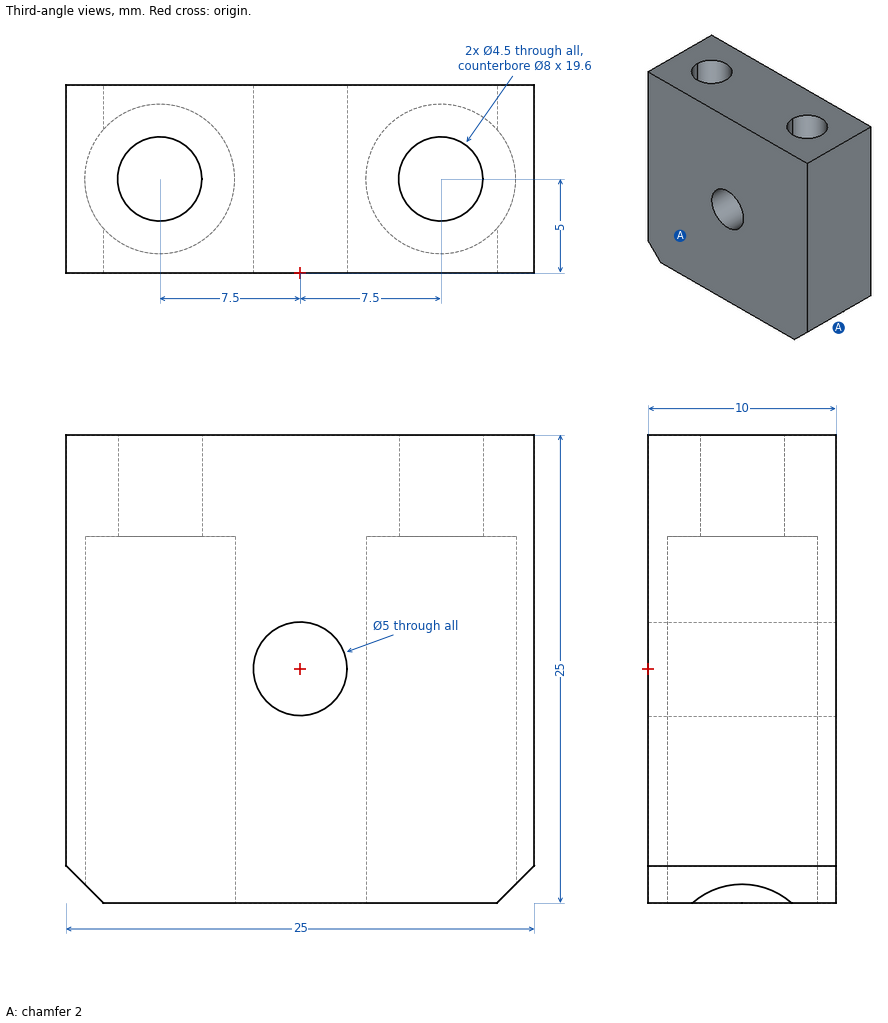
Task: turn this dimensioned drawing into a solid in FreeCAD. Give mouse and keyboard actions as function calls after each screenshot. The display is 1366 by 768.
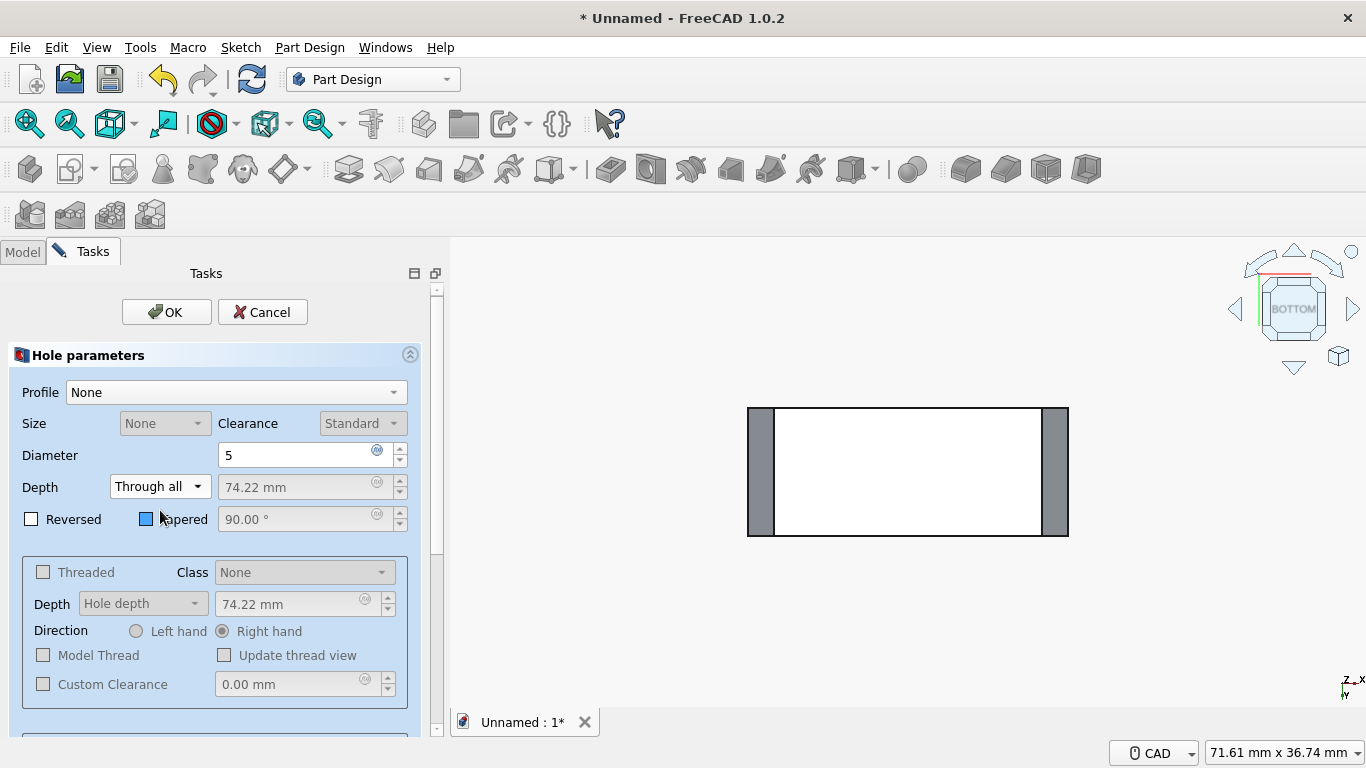
click(167, 312)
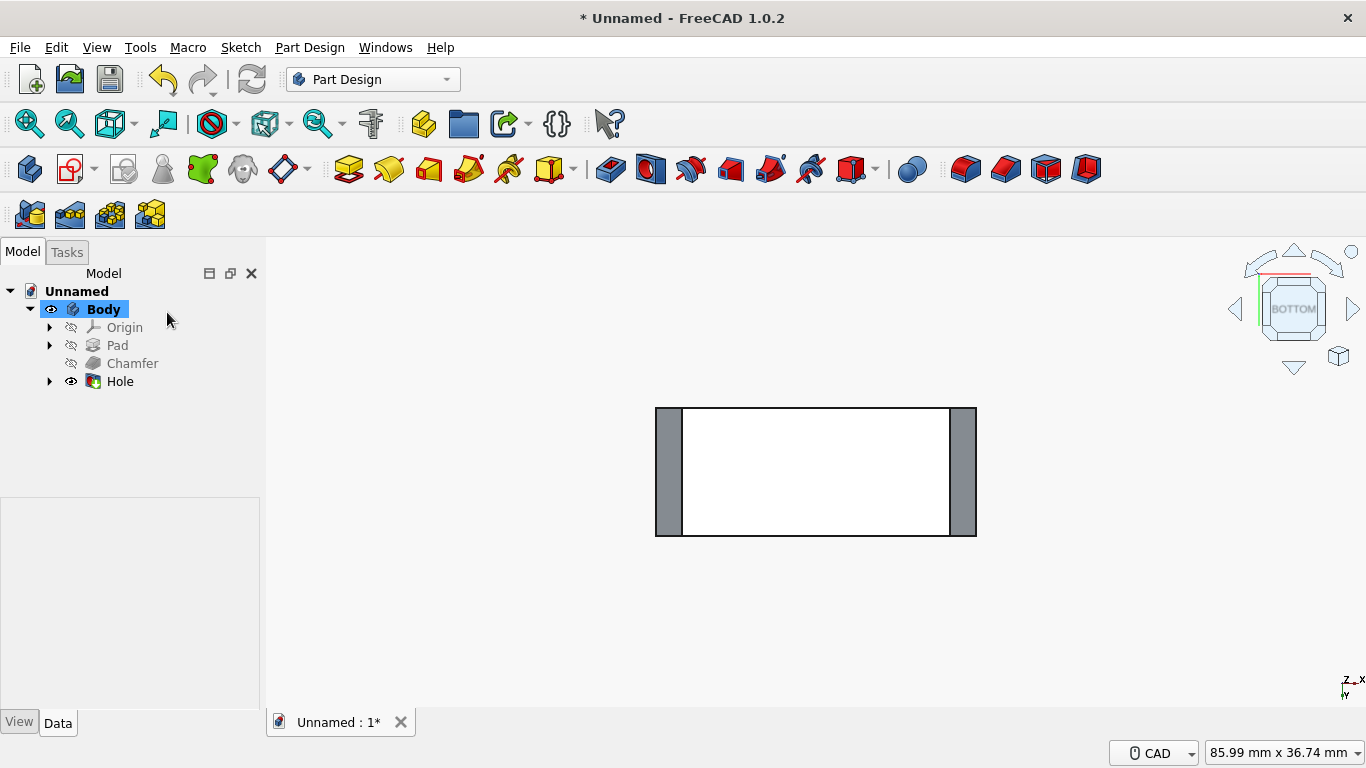
click(30, 124)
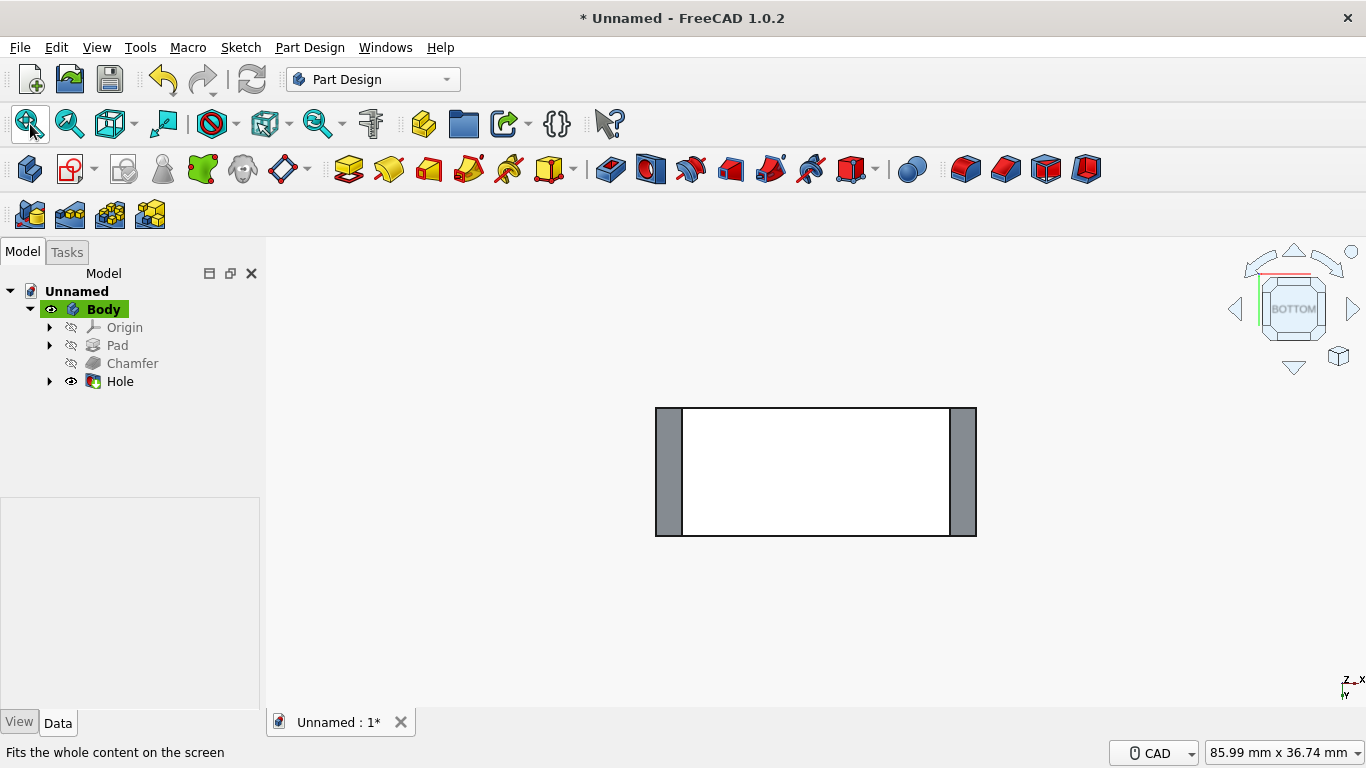
click(854, 471)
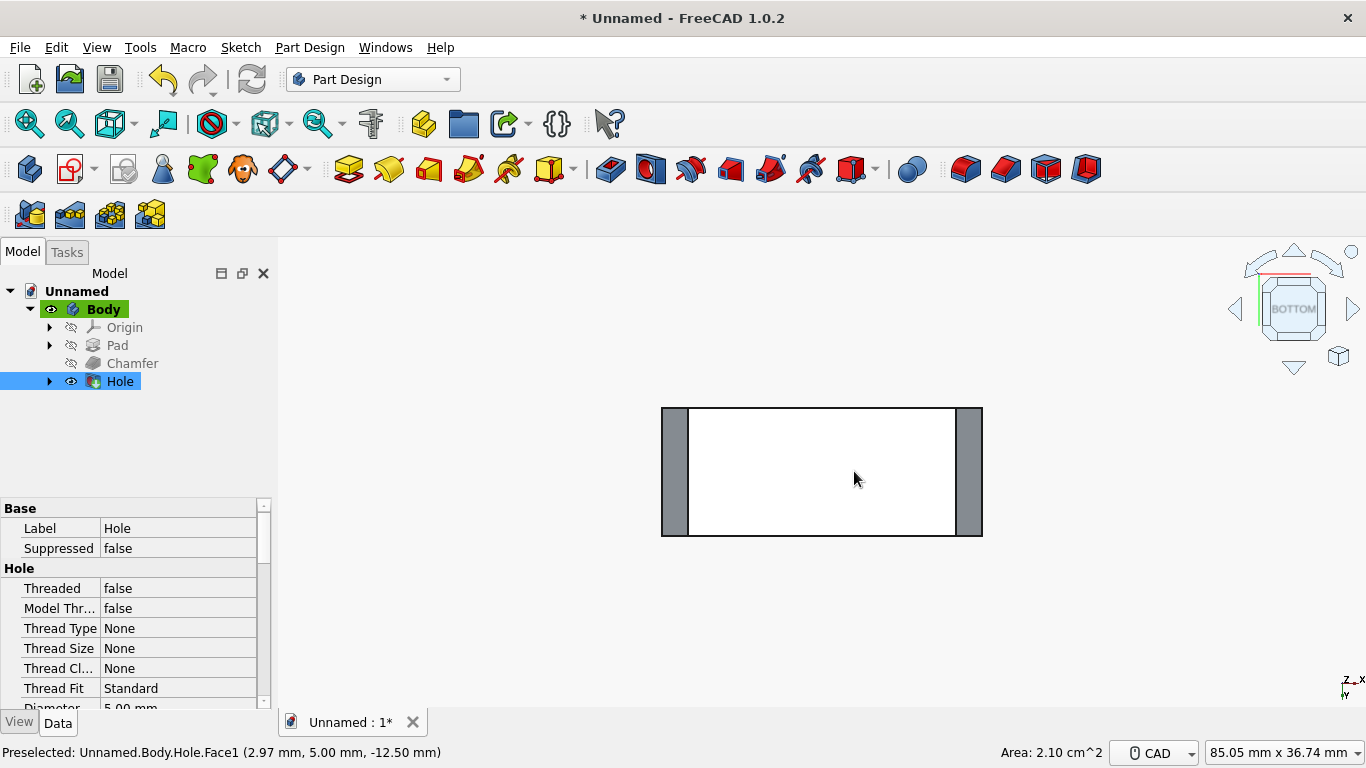
click(70, 170)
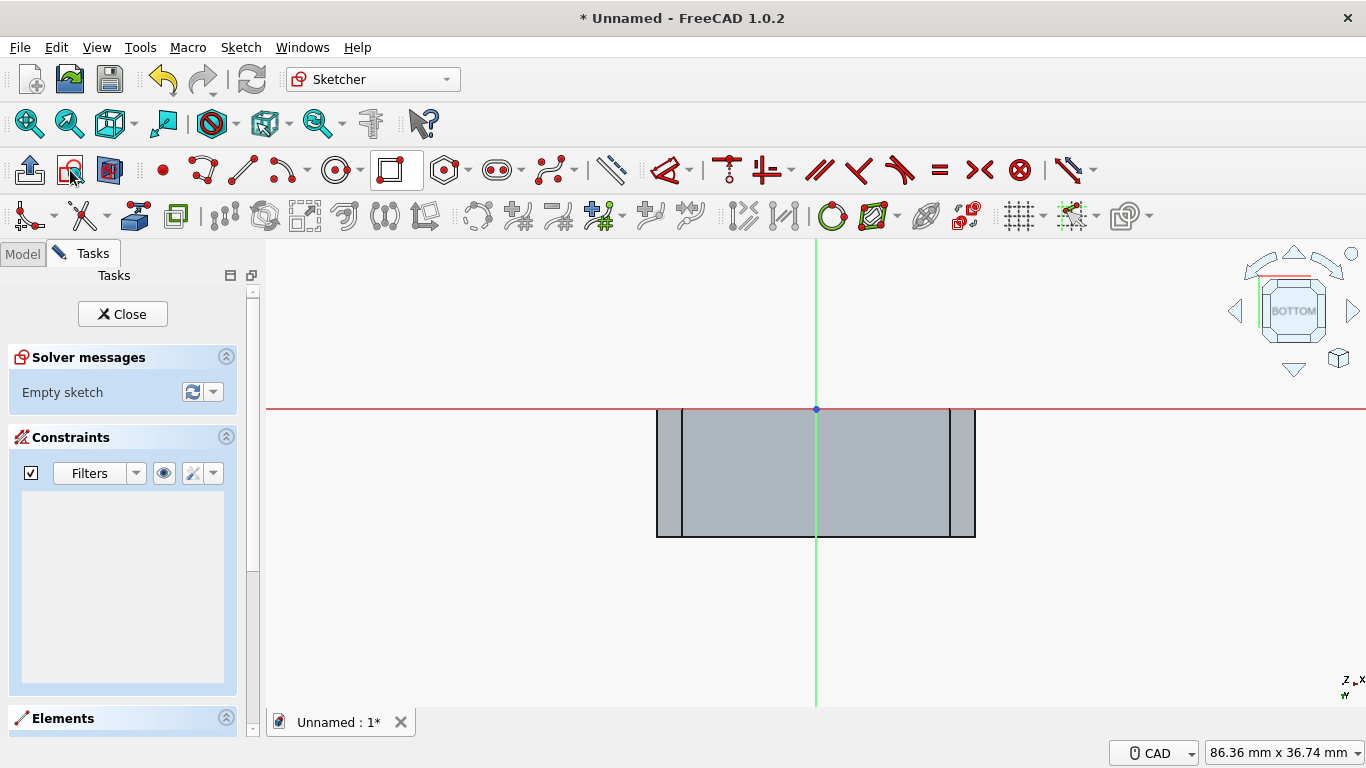
scroll(856, 445, up, 5)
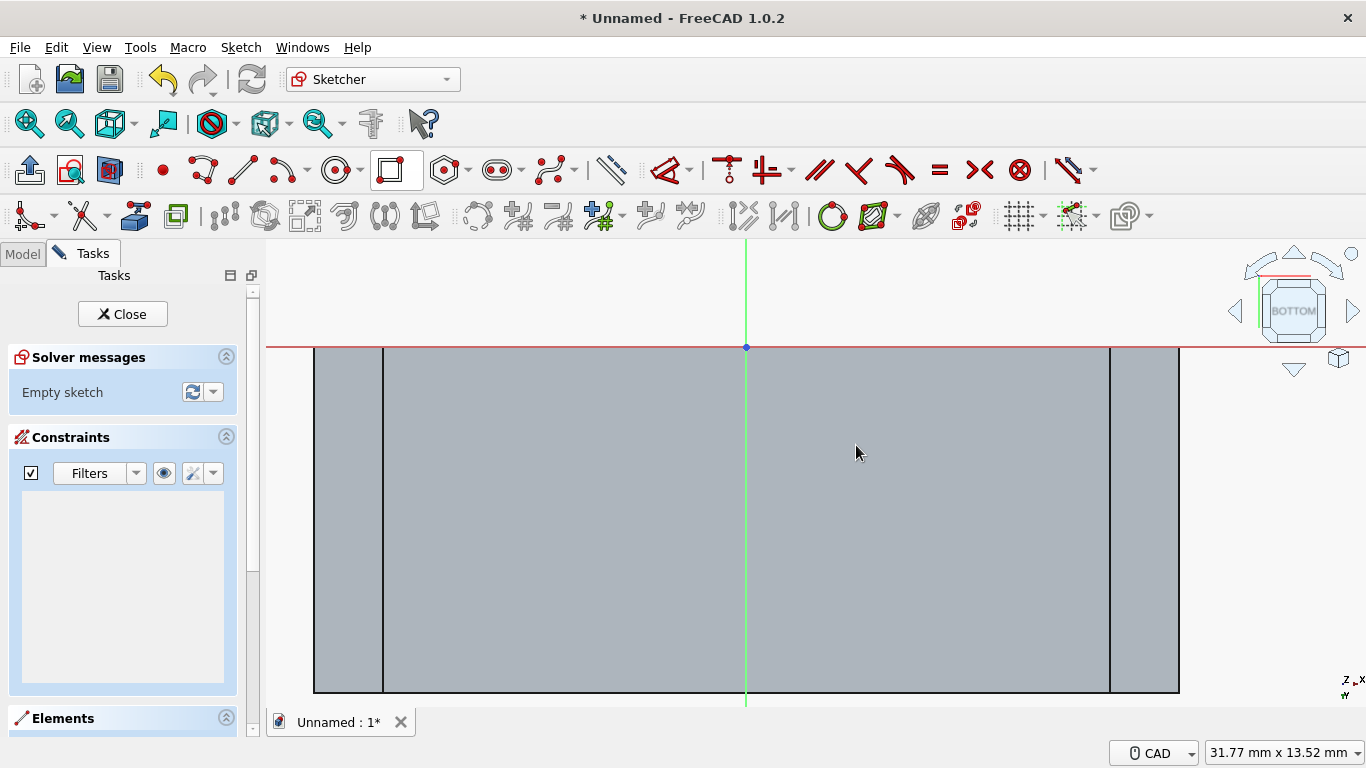
key(g)
key(c)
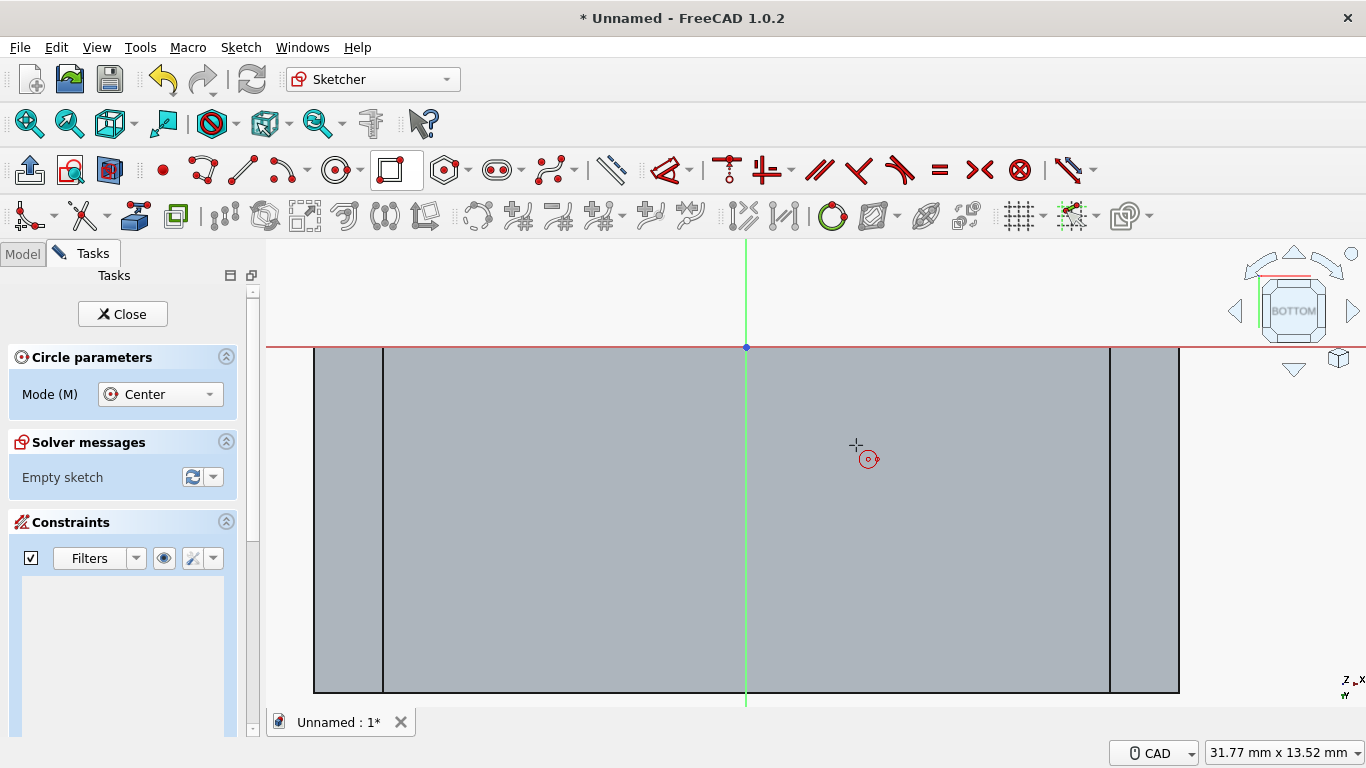
click(1006, 520)
move(1061, 465)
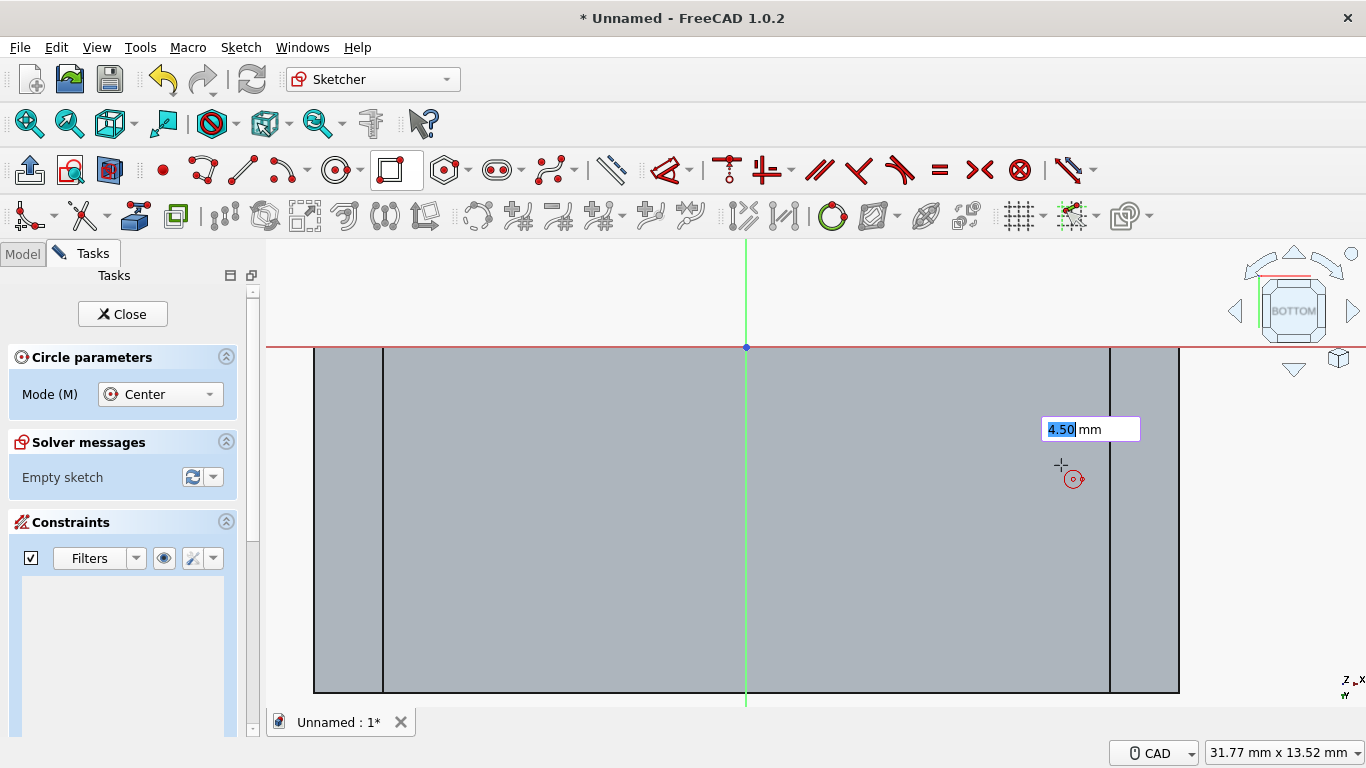
text(4.5)
key(Return)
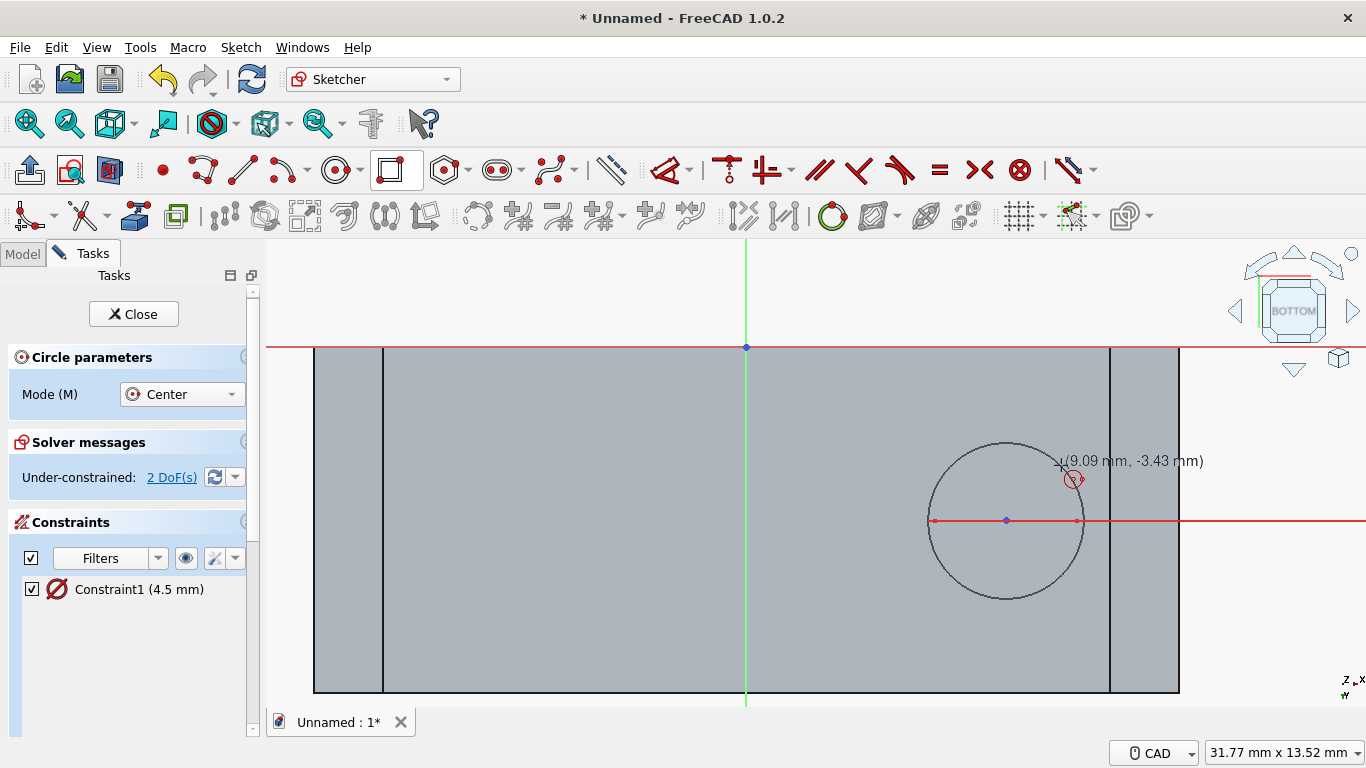
click(487, 520)
move(542, 465)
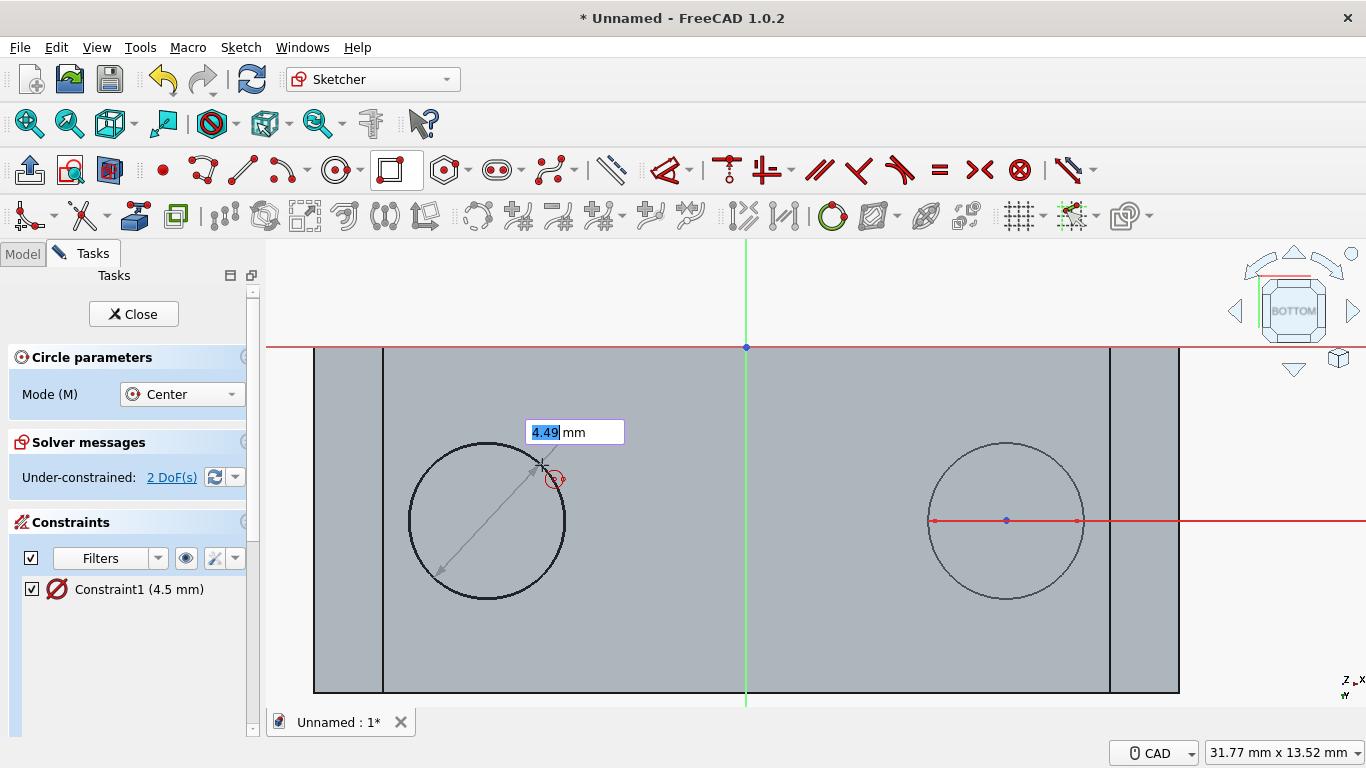
text(4.5)
key(Return)
key(Escape)